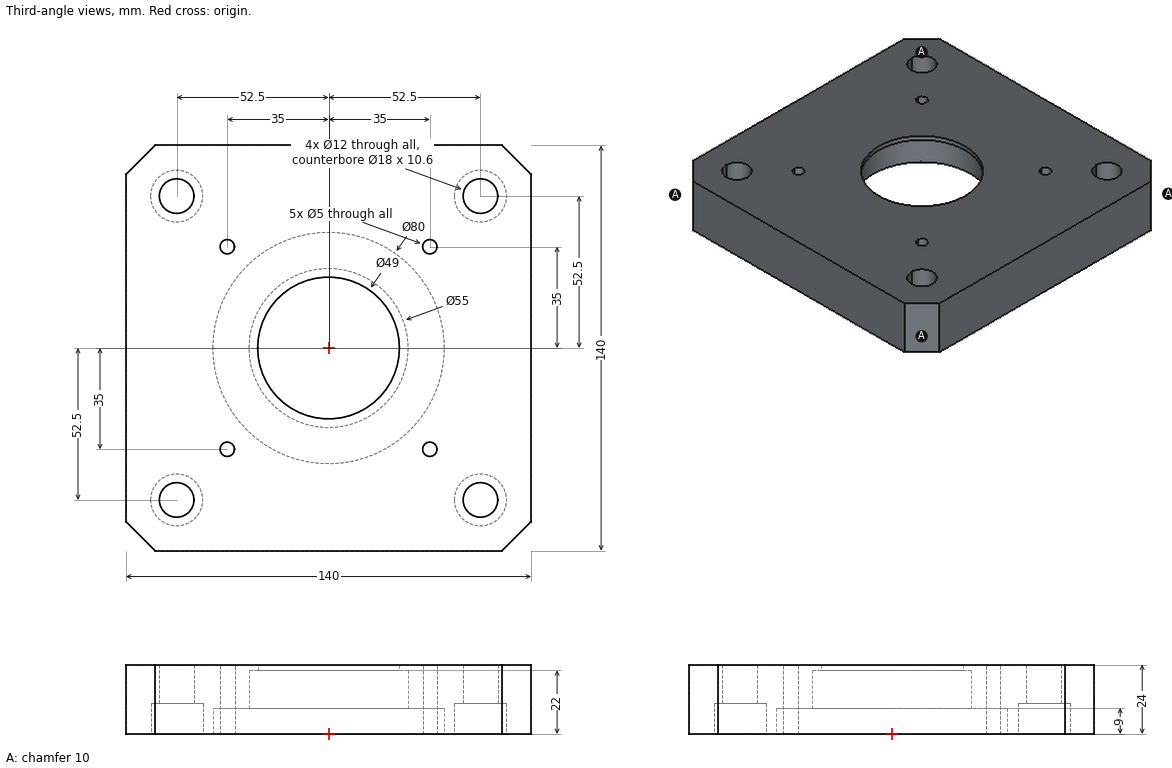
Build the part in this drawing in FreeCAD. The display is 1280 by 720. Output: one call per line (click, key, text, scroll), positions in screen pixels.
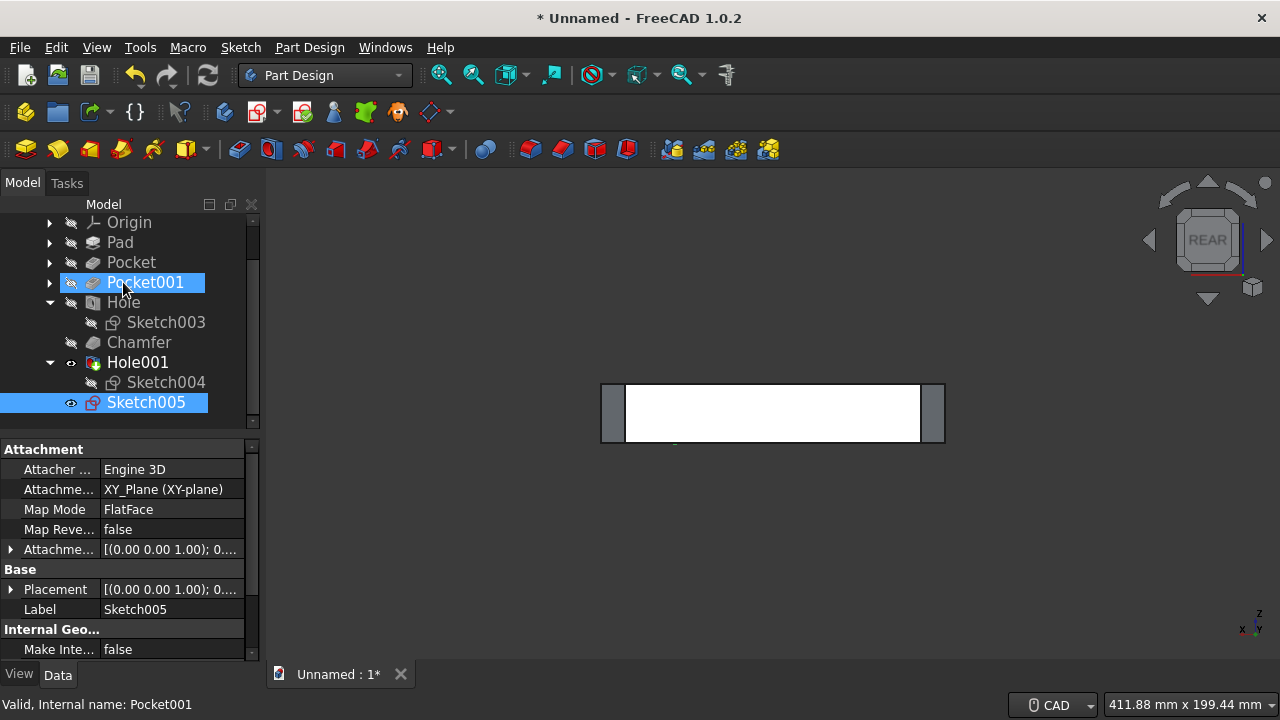
click(240, 150)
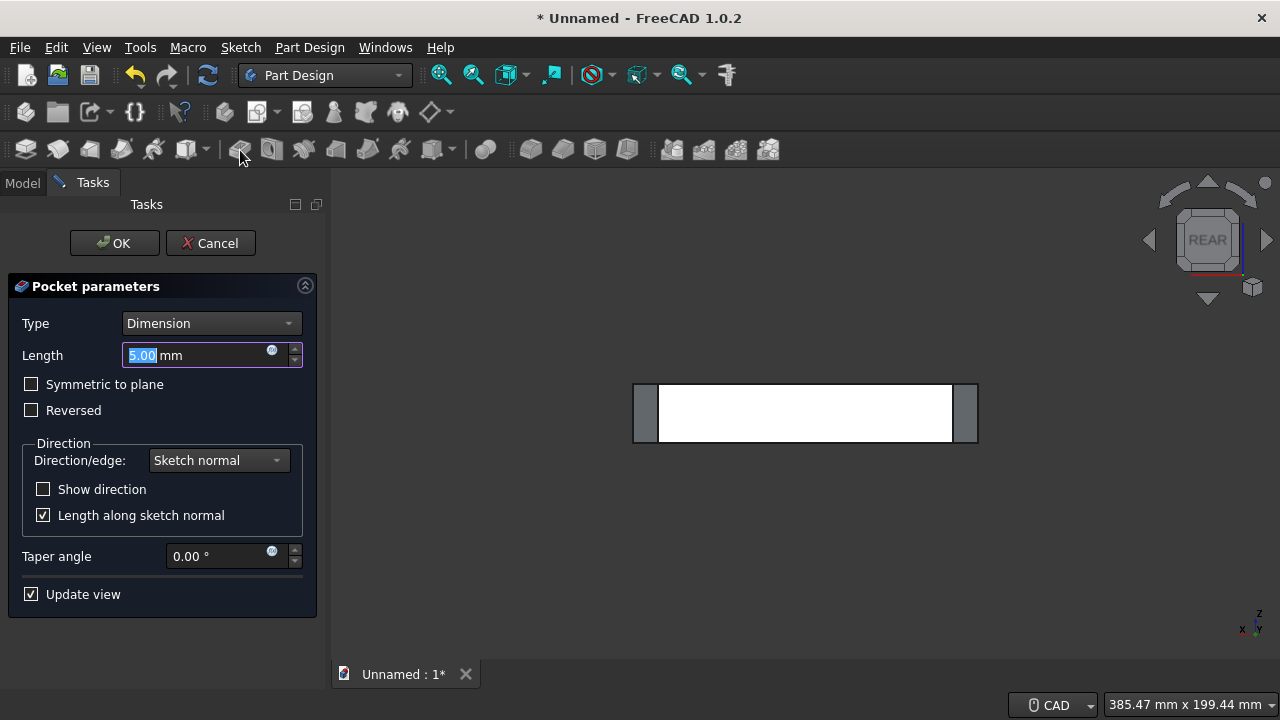
text(9)
key(Tab)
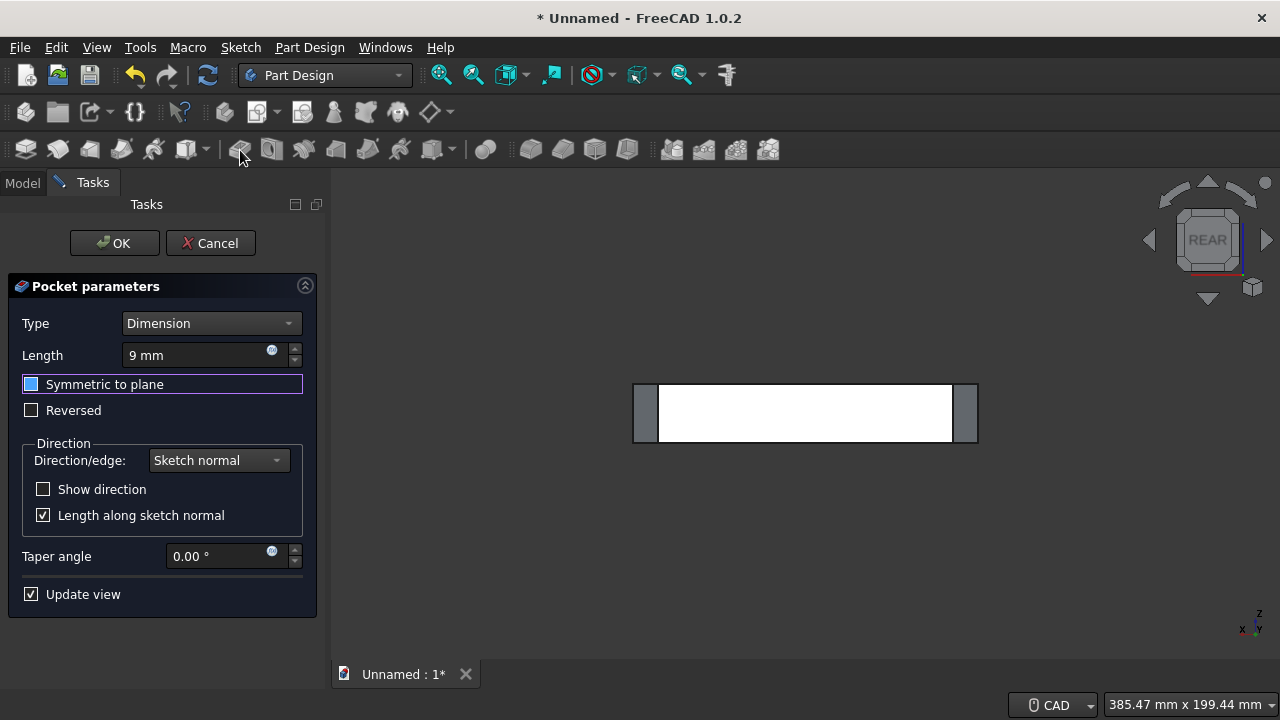
click(30, 410)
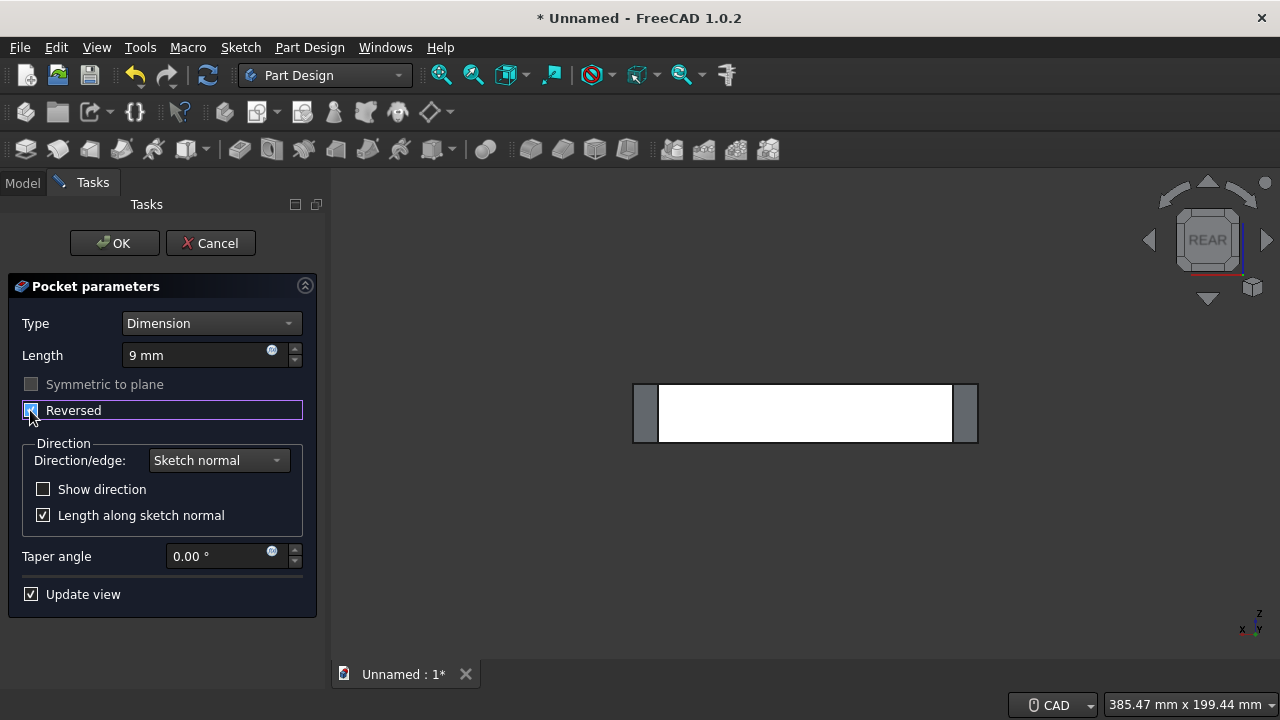
click(115, 243)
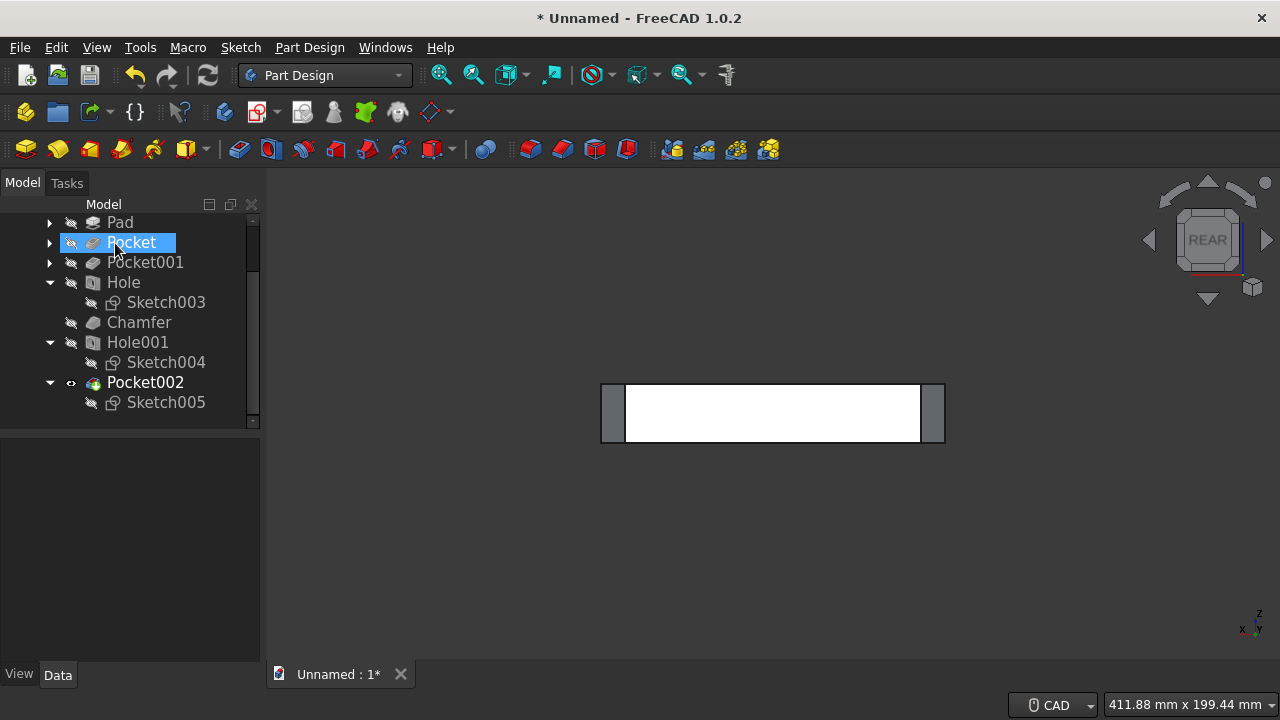
key(0)